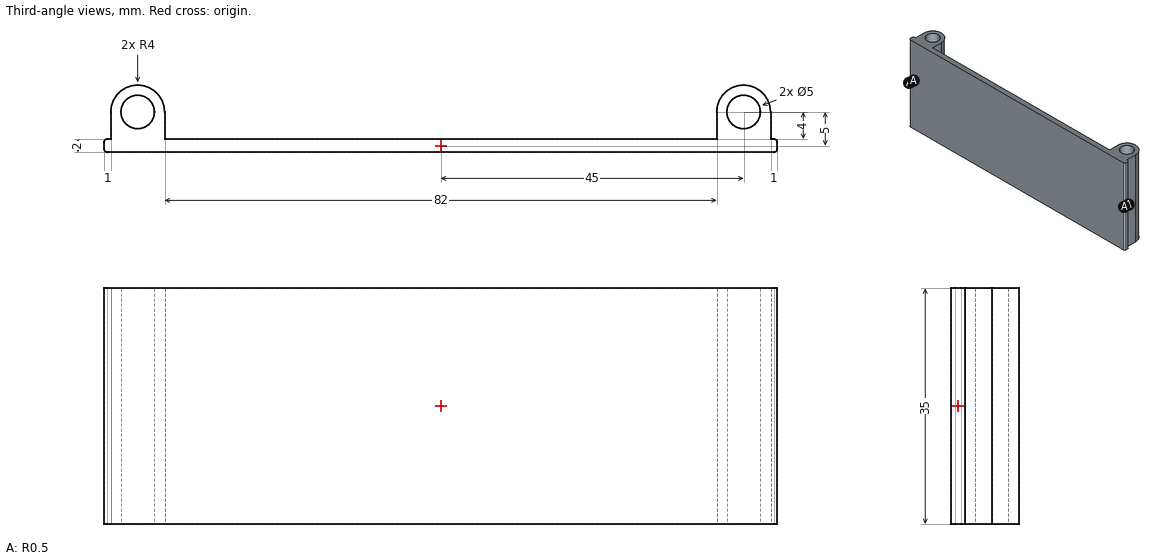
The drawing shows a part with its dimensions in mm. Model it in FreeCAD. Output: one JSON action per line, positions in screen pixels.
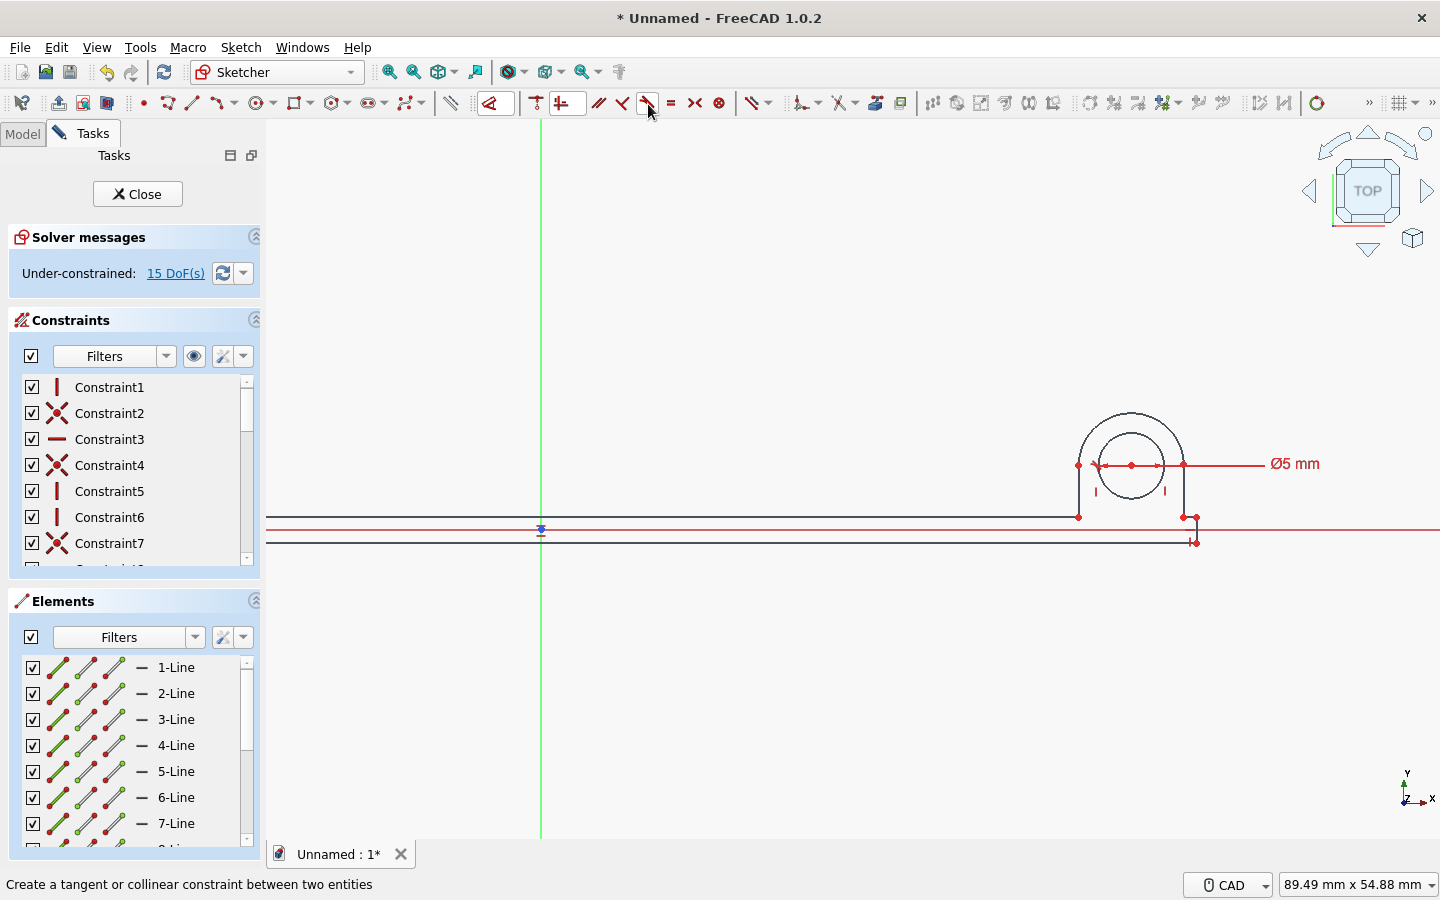
{"action": "scroll", "coordinate": [1080, 481], "scroll_direction": "down", "scroll_amount": 3}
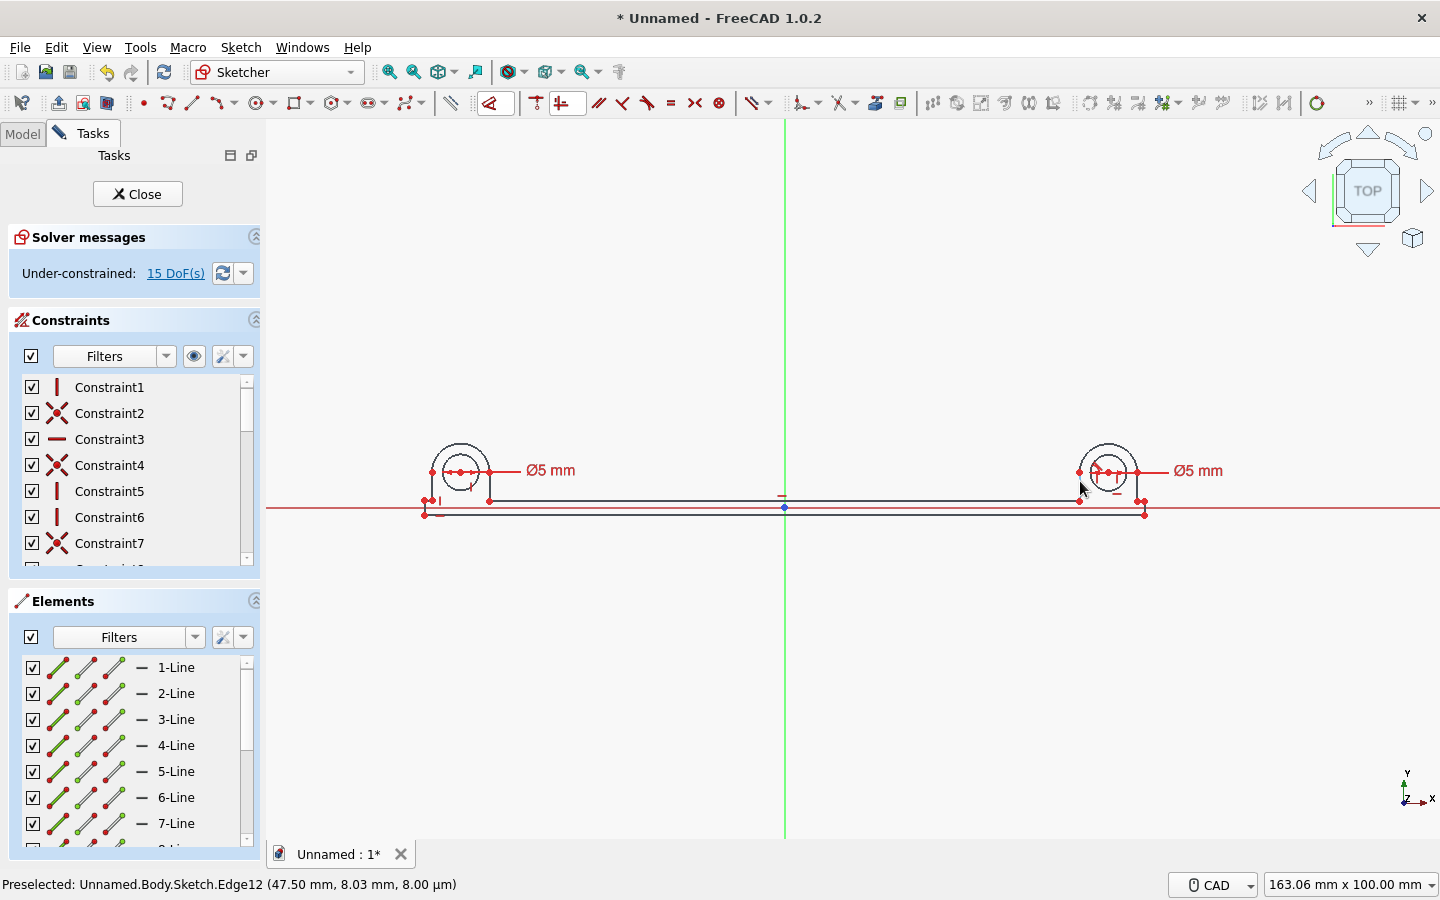
{"action": "scroll", "coordinate": [490, 492], "scroll_direction": "up", "scroll_amount": 3}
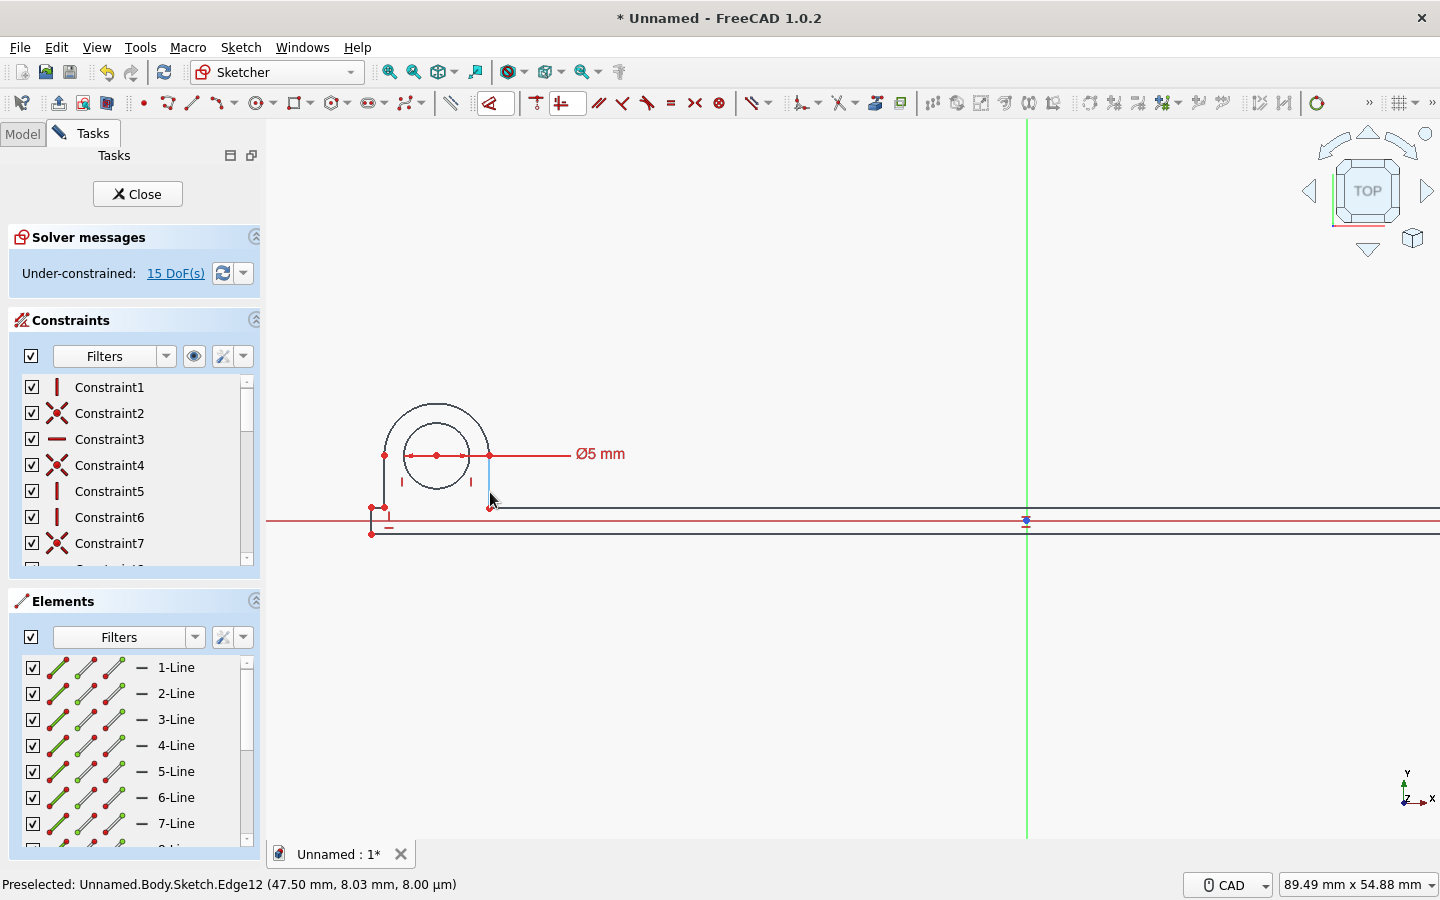
{"action": "left_click", "coordinate": [489, 492]}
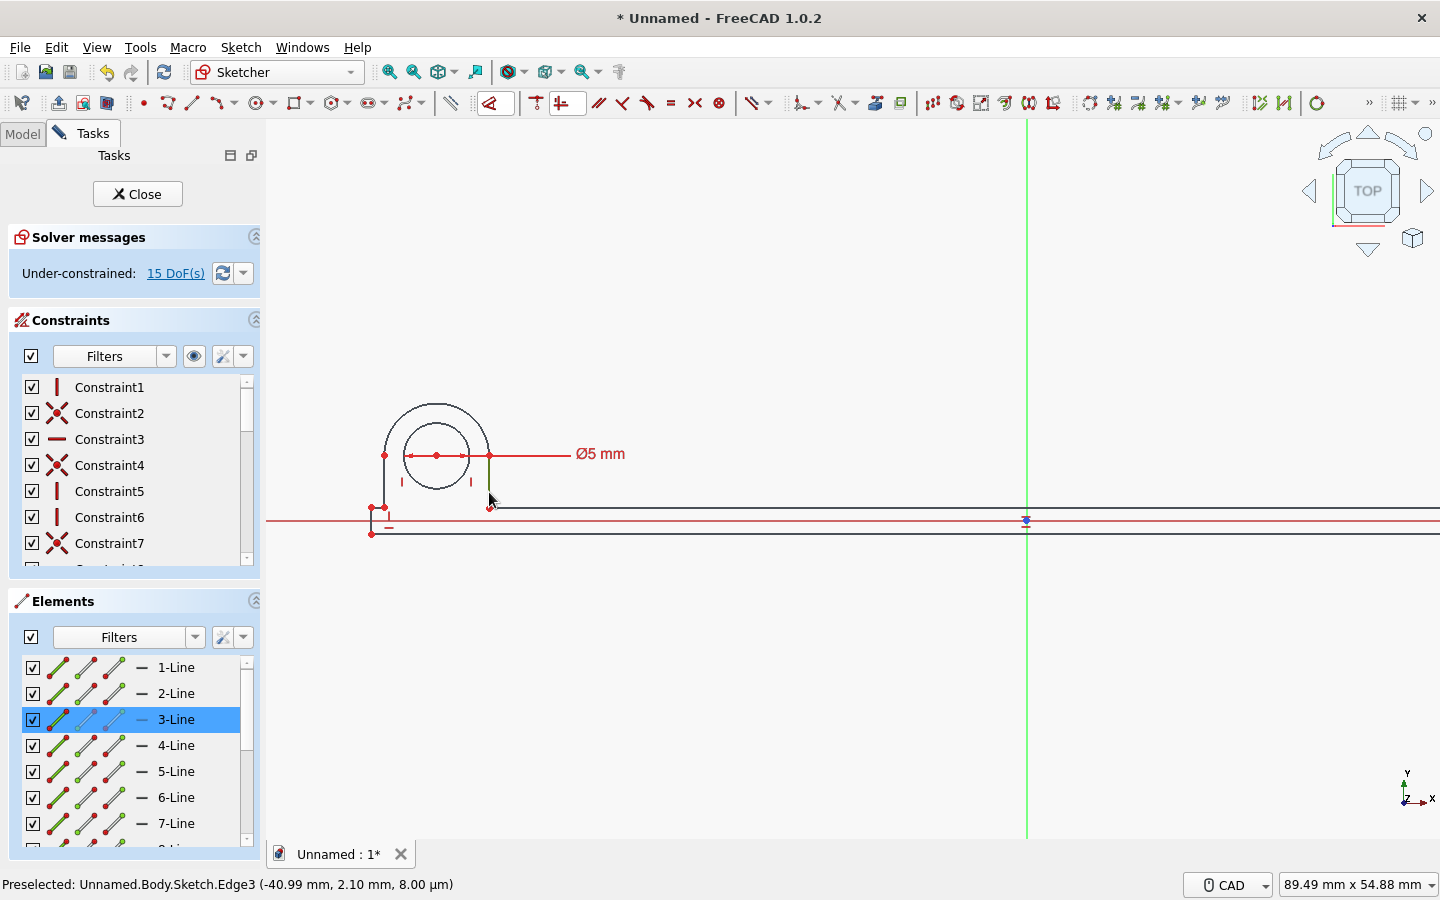
{"action": "left_click", "coordinate": [467, 413]}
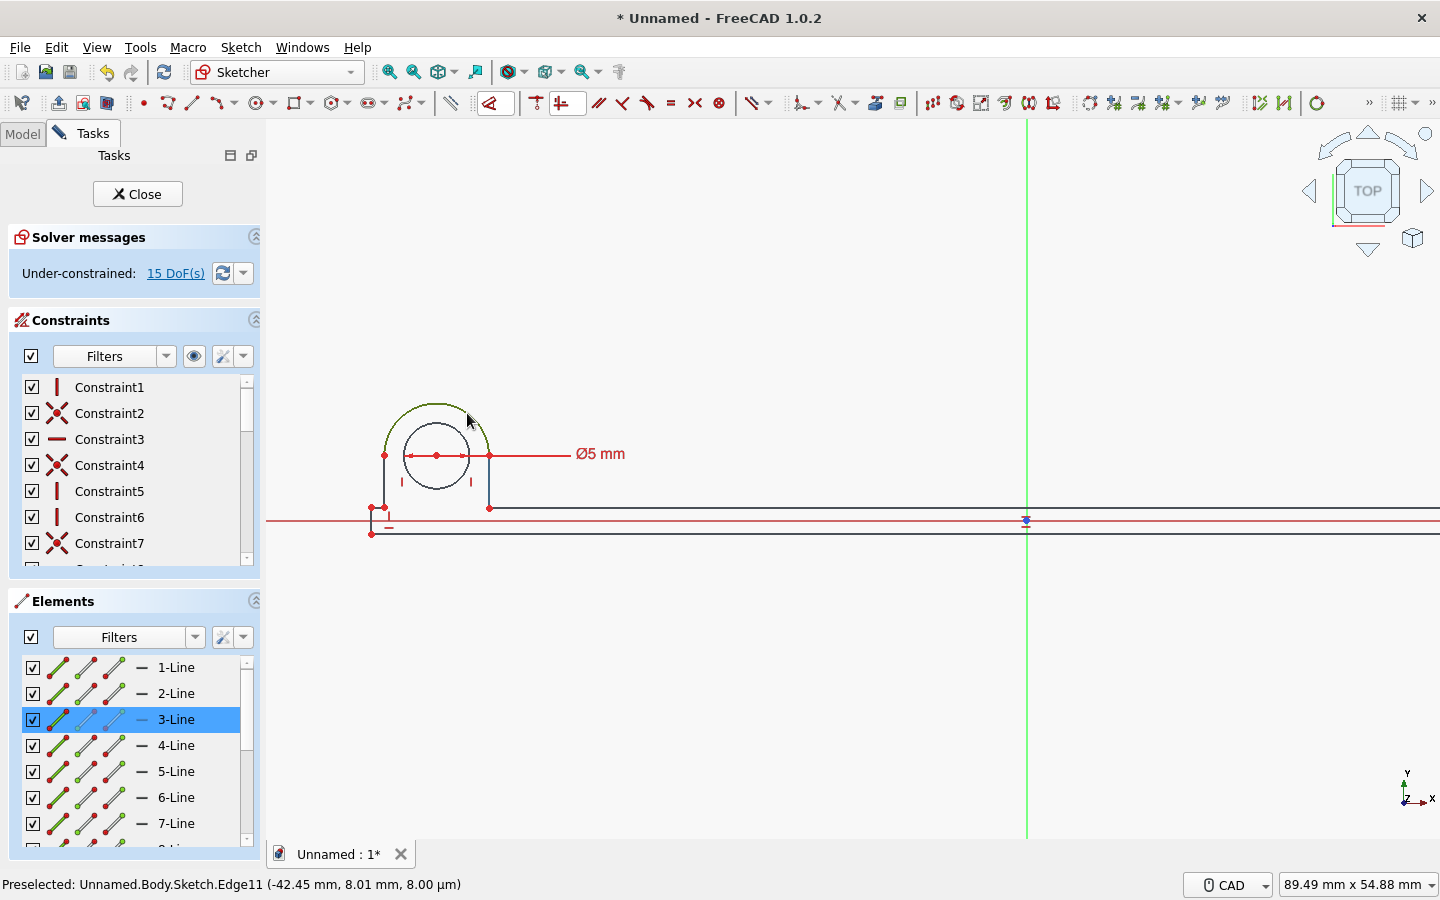
{"action": "left_click", "coordinate": [648, 104]}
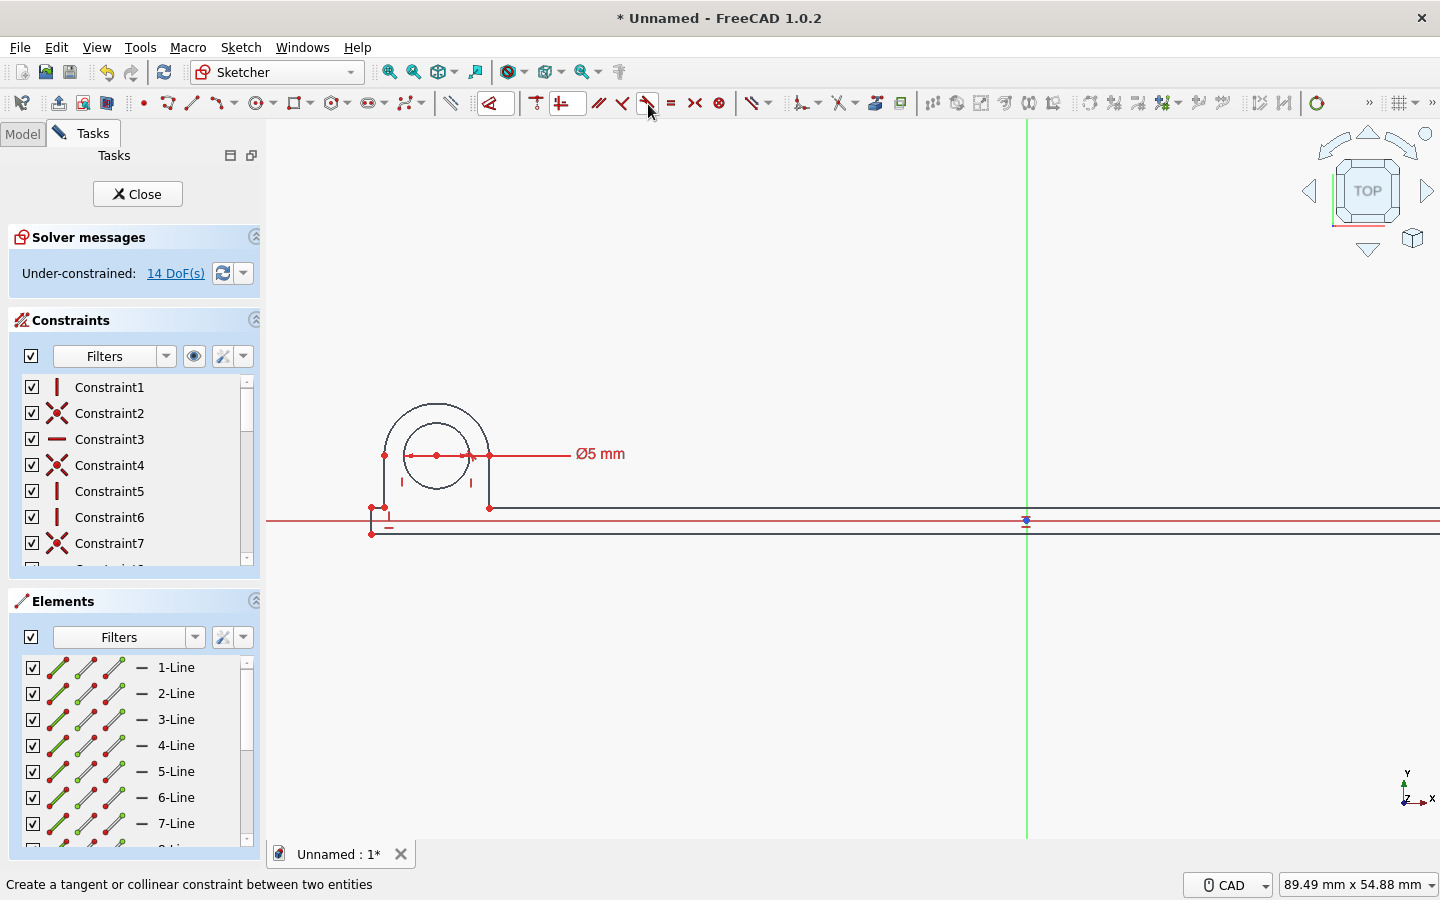
{"action": "left_click", "coordinate": [384, 471]}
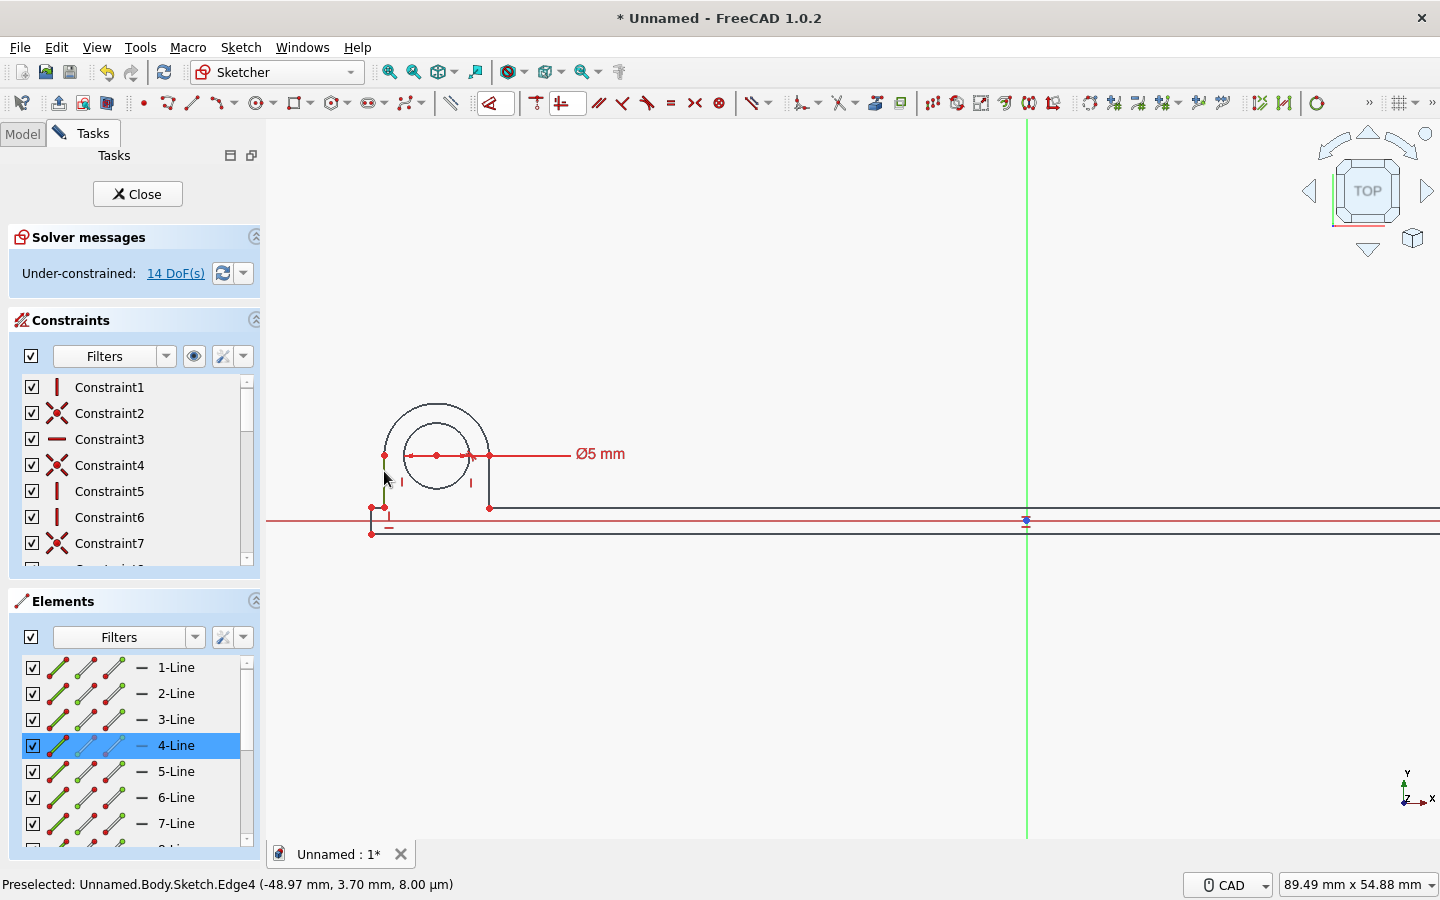
{"action": "left_click", "coordinate": [468, 414]}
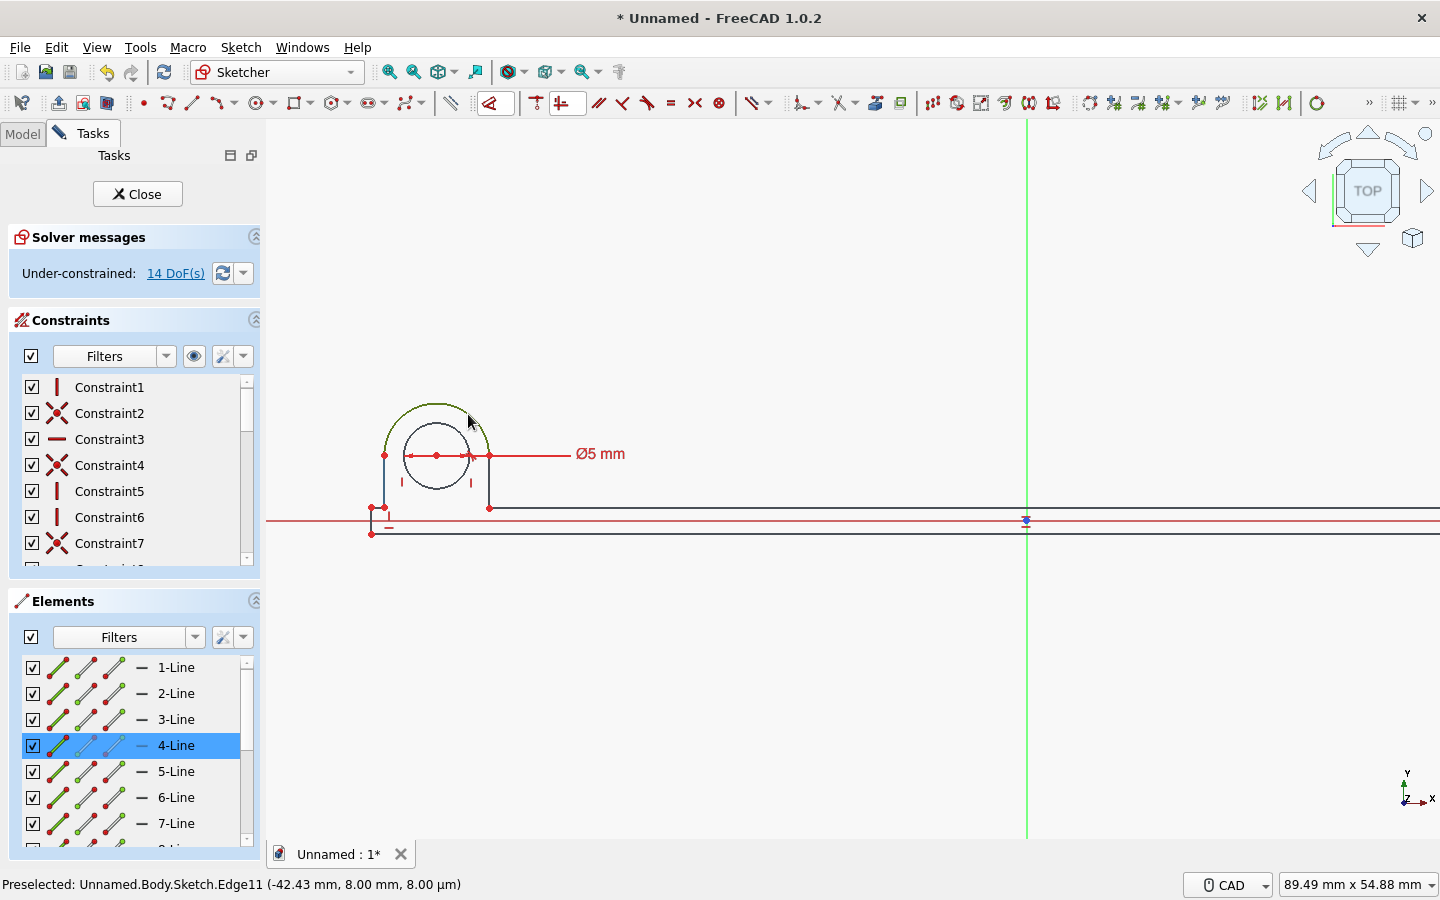
{"action": "key", "text": "t"}